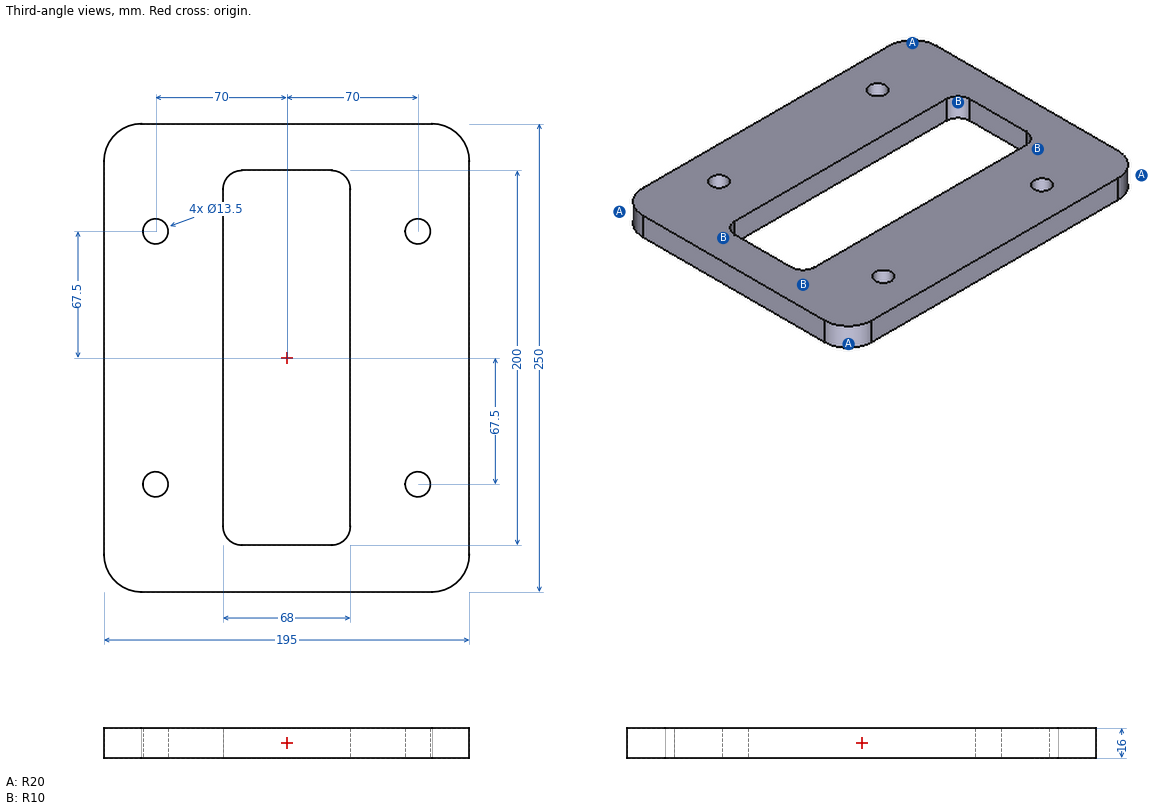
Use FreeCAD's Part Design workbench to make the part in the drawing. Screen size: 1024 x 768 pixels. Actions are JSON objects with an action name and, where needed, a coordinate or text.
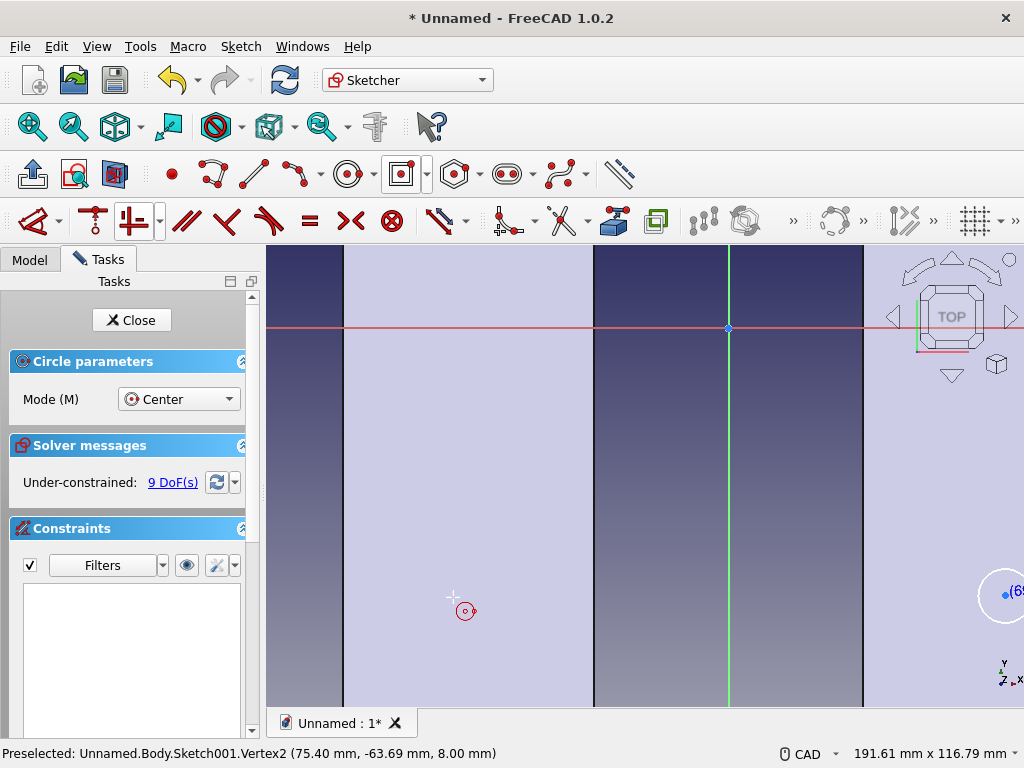
{"action": "left_click", "coordinate": [452, 595]}
{"action": "left_click", "coordinate": [471, 576]}
{"action": "key", "text": "Escape"}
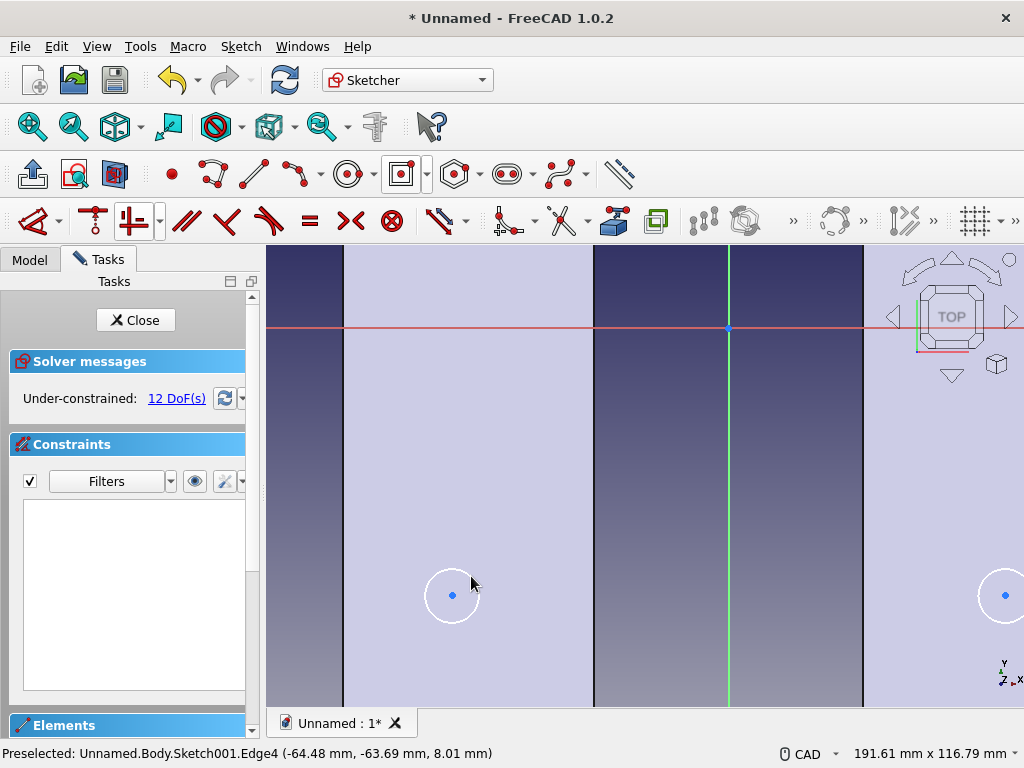
{"action": "scroll", "coordinate": [452, 597], "scroll_direction": "down", "scroll_amount": 4}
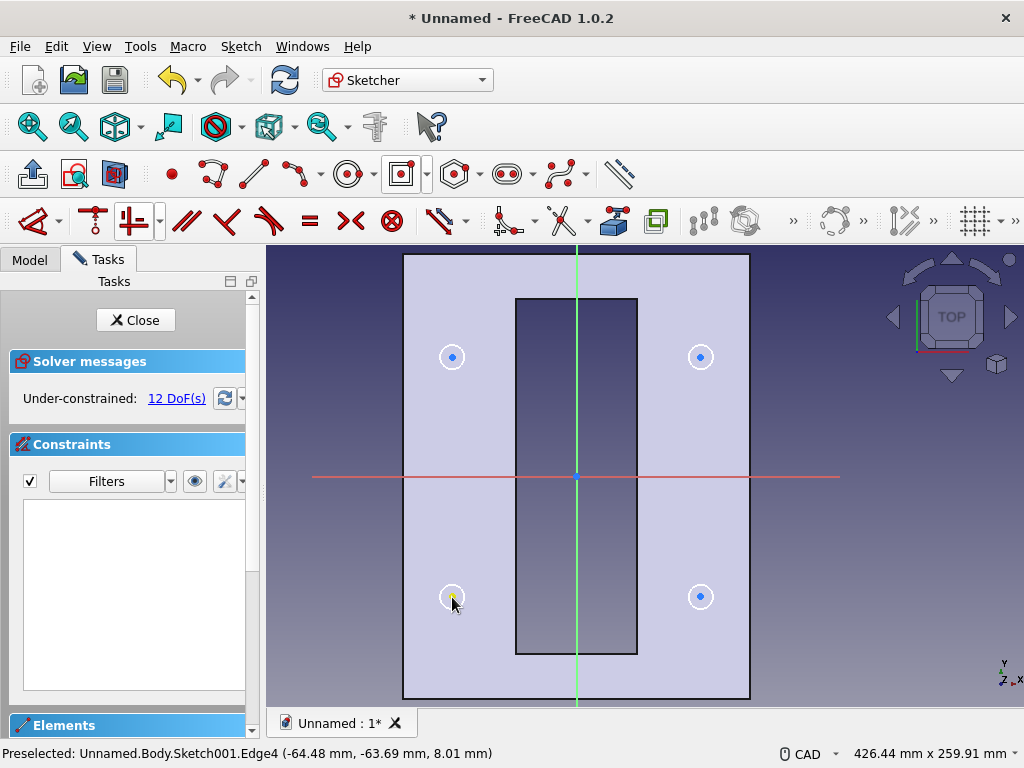
{"action": "left_click", "coordinate": [461, 349]}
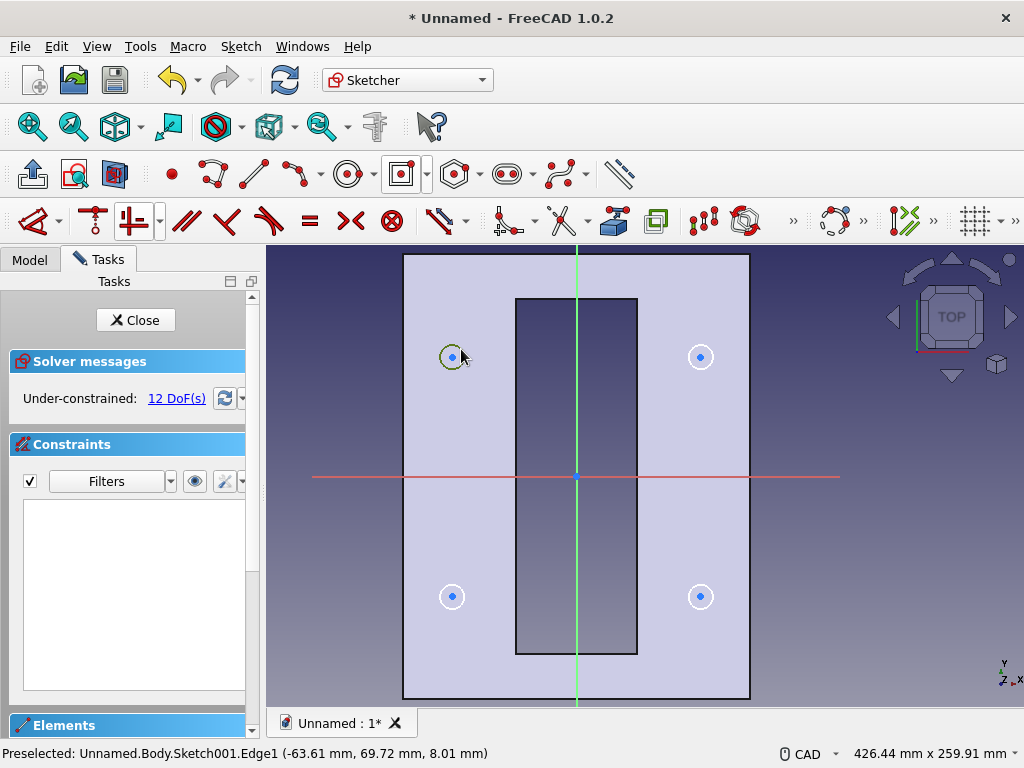
{"action": "left_click", "coordinate": [709, 349]}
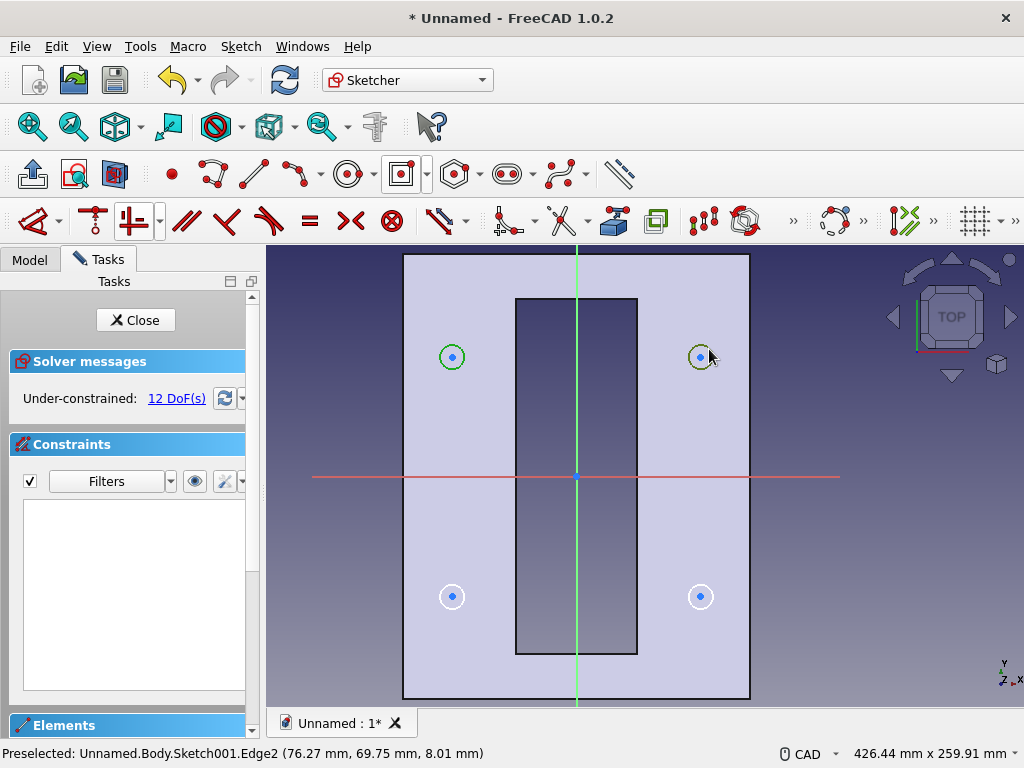
{"action": "left_click", "coordinate": [709, 588]}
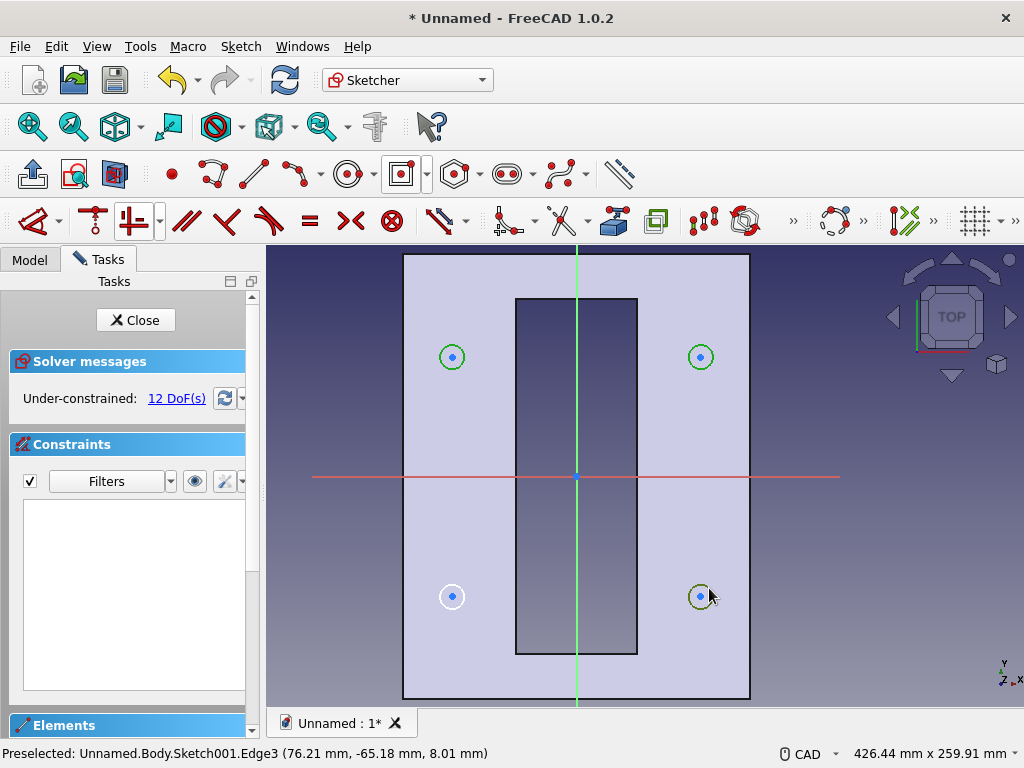
{"action": "left_click", "coordinate": [461, 588]}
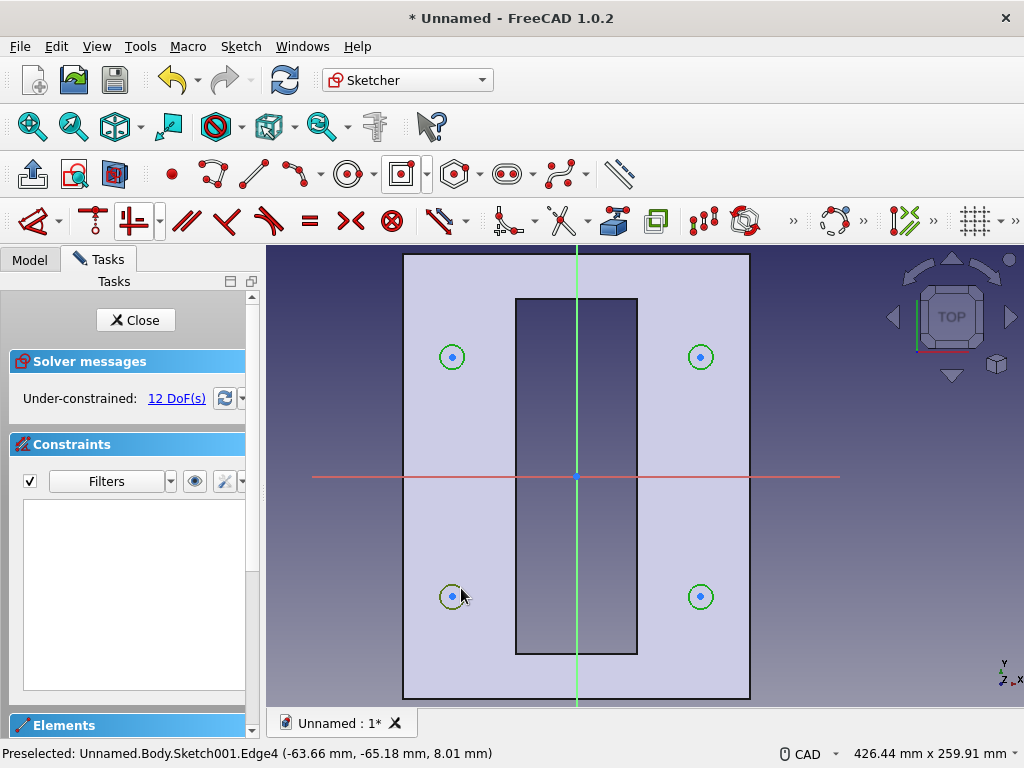
{"action": "left_click", "coordinate": [310, 222]}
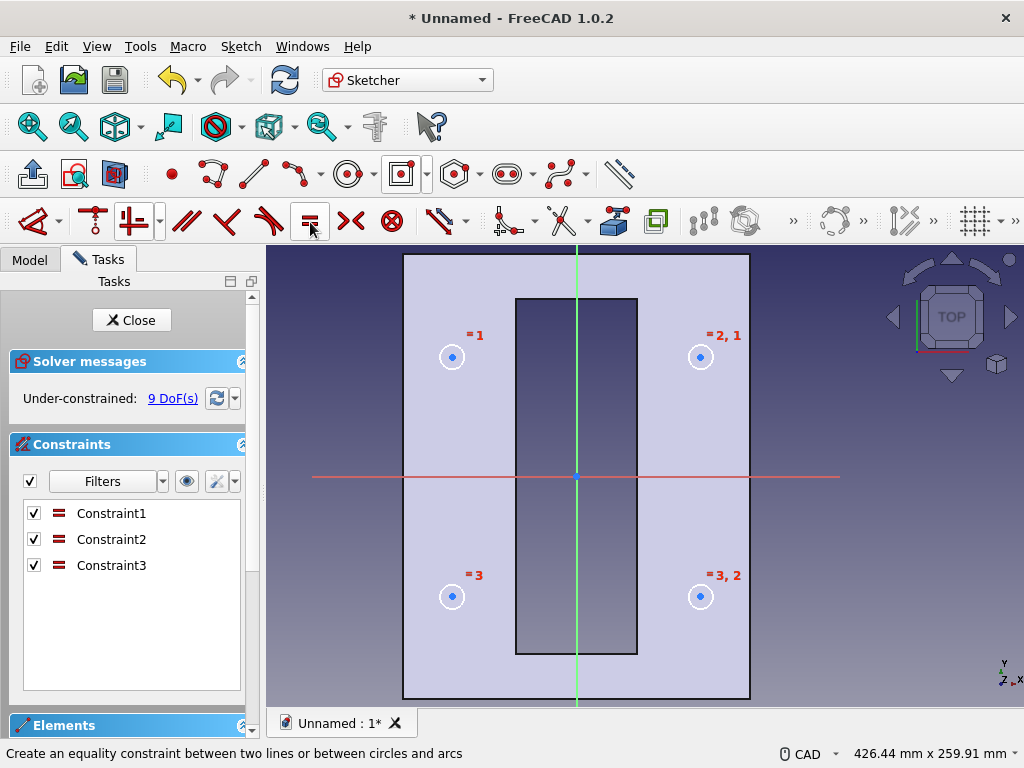
{"action": "left_click", "coordinate": [452, 357]}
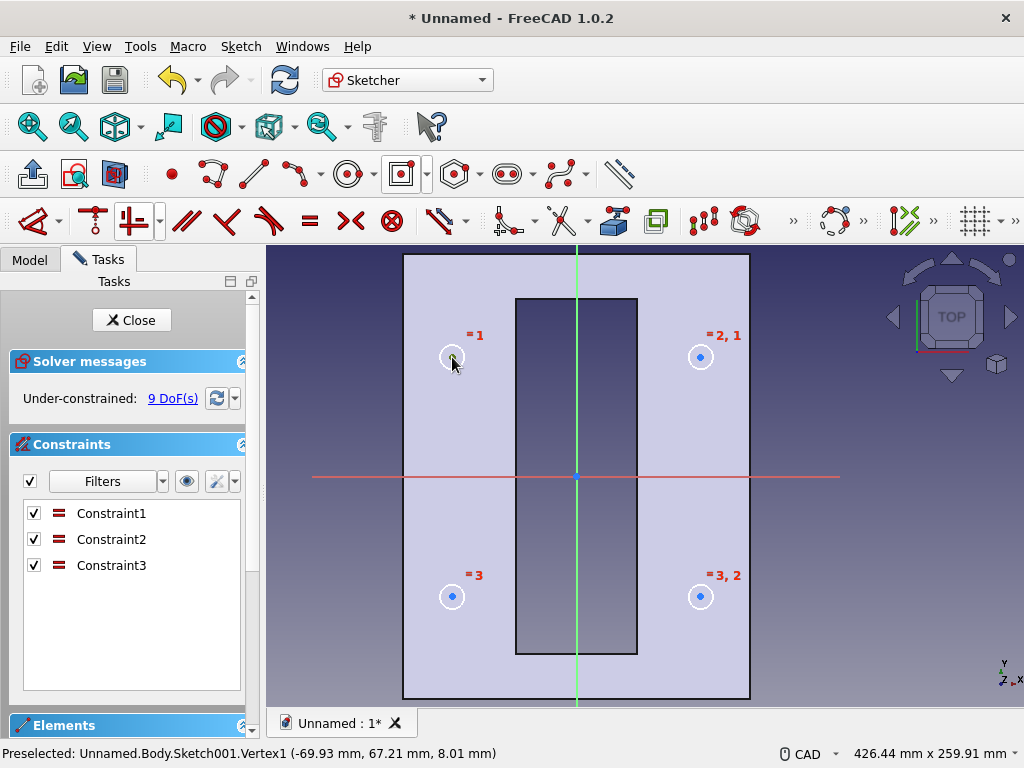
{"action": "left_click", "coordinate": [701, 357]}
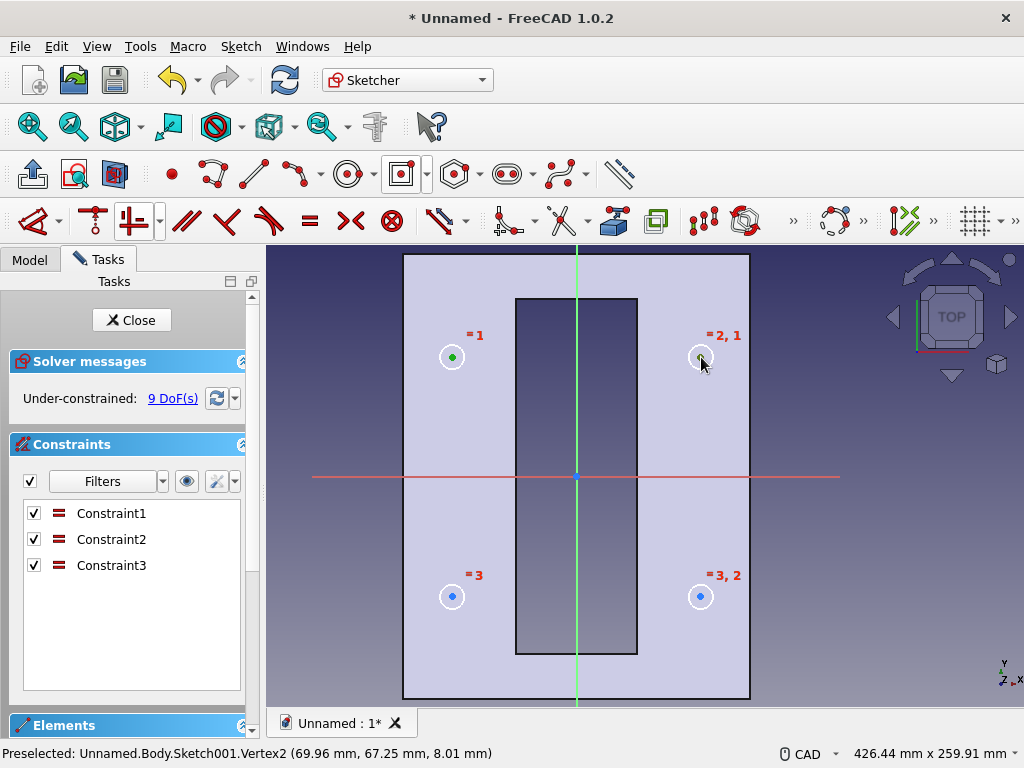
{"action": "left_click", "coordinate": [160, 222]}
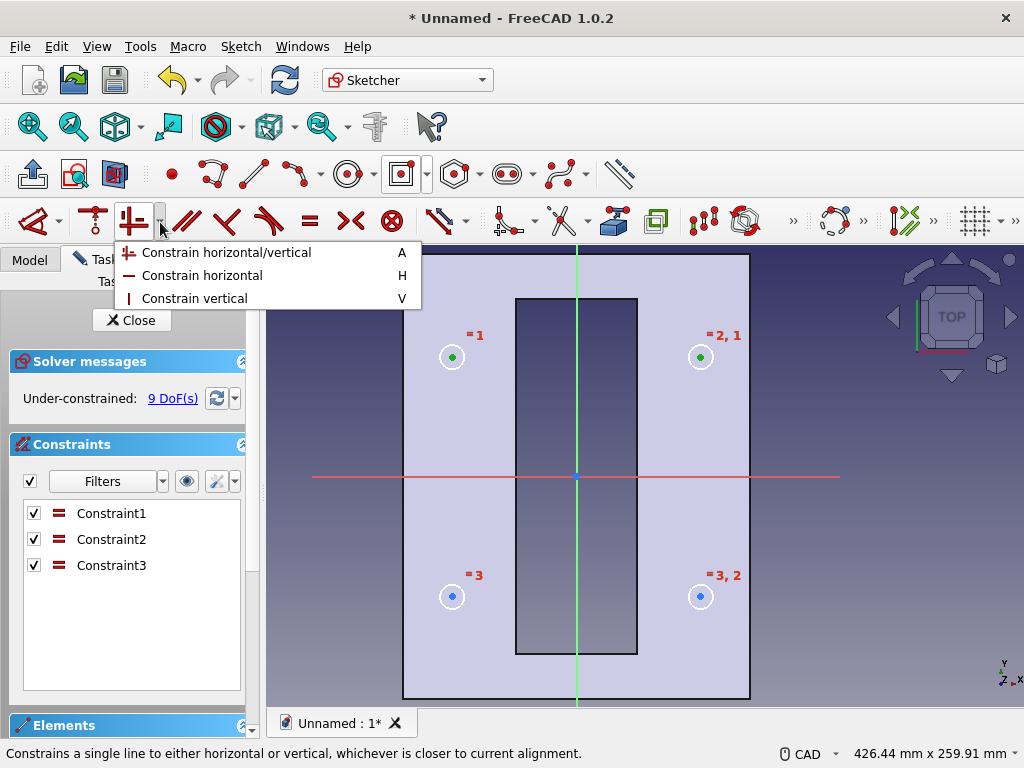
{"action": "left_click", "coordinate": [268, 276]}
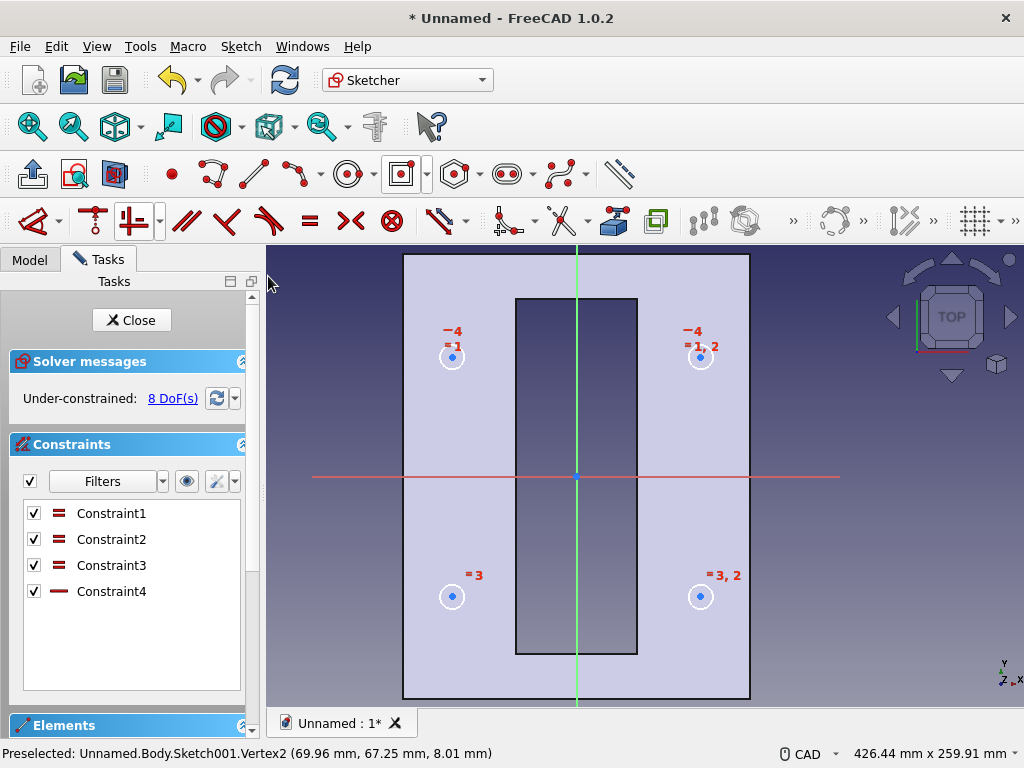
{"action": "left_click", "coordinate": [701, 357]}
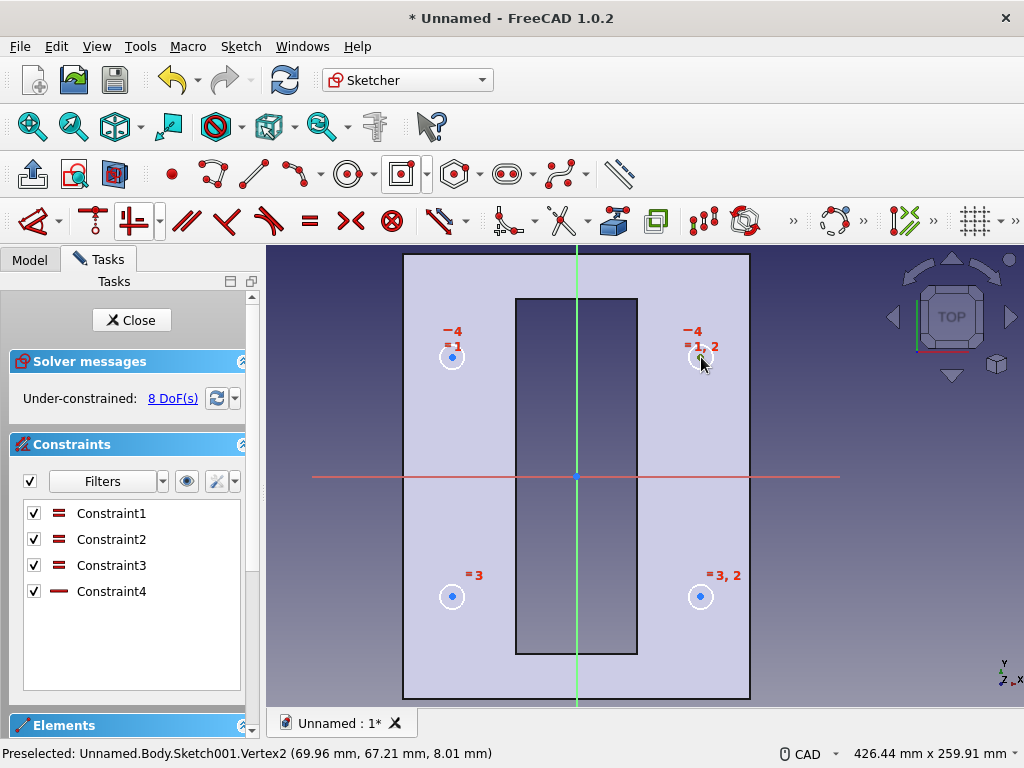
{"action": "left_click", "coordinate": [701, 597]}